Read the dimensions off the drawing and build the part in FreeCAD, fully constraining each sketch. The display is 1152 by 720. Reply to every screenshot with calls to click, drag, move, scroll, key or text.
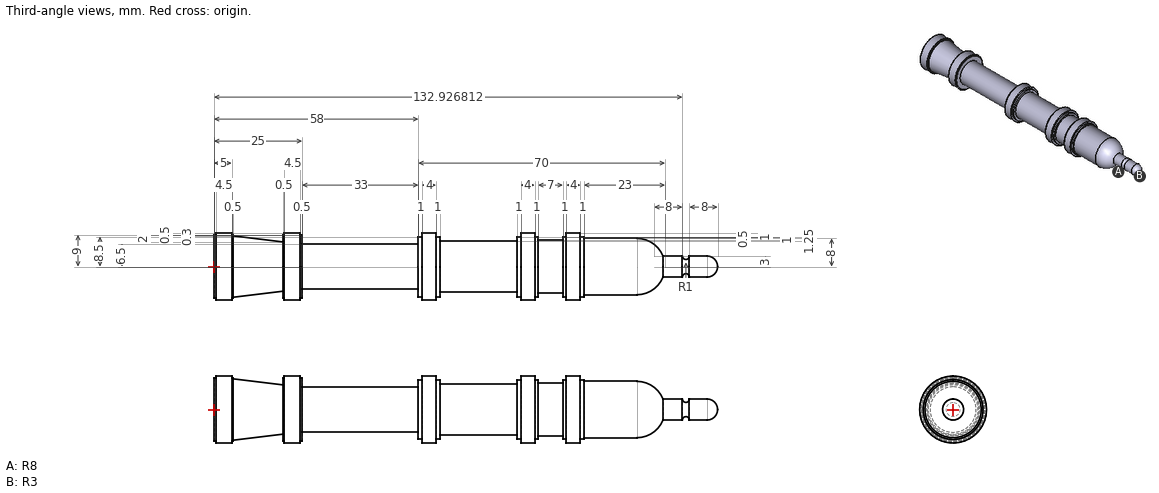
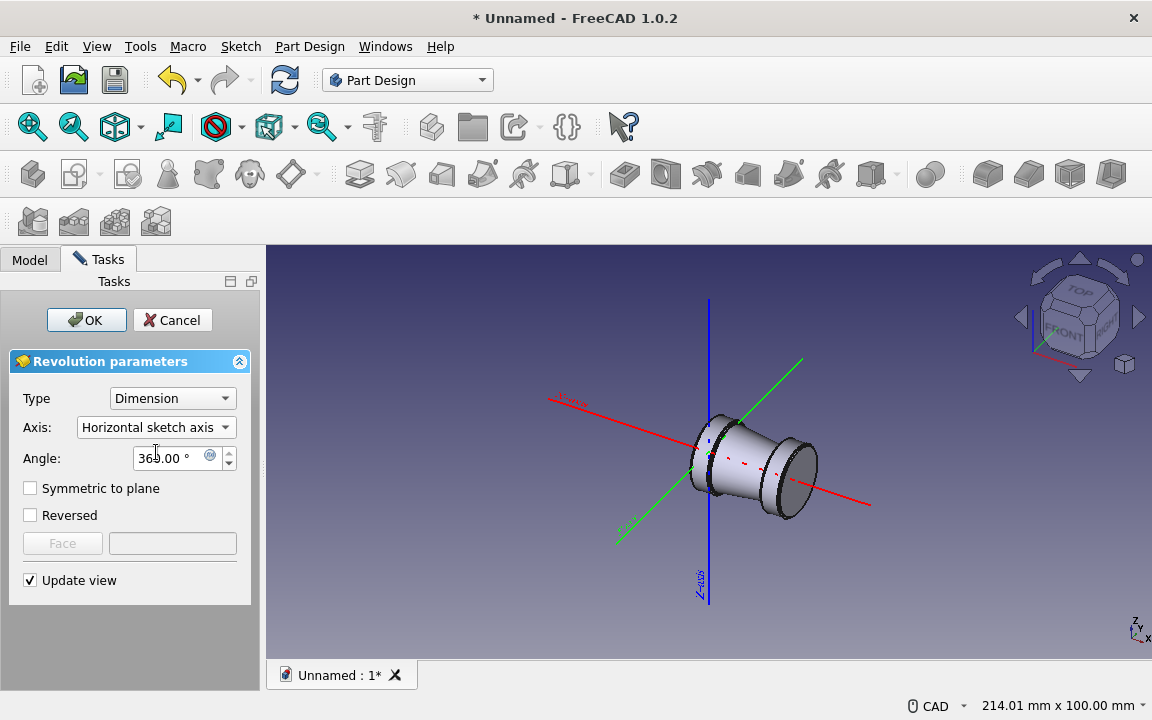
click(87, 320)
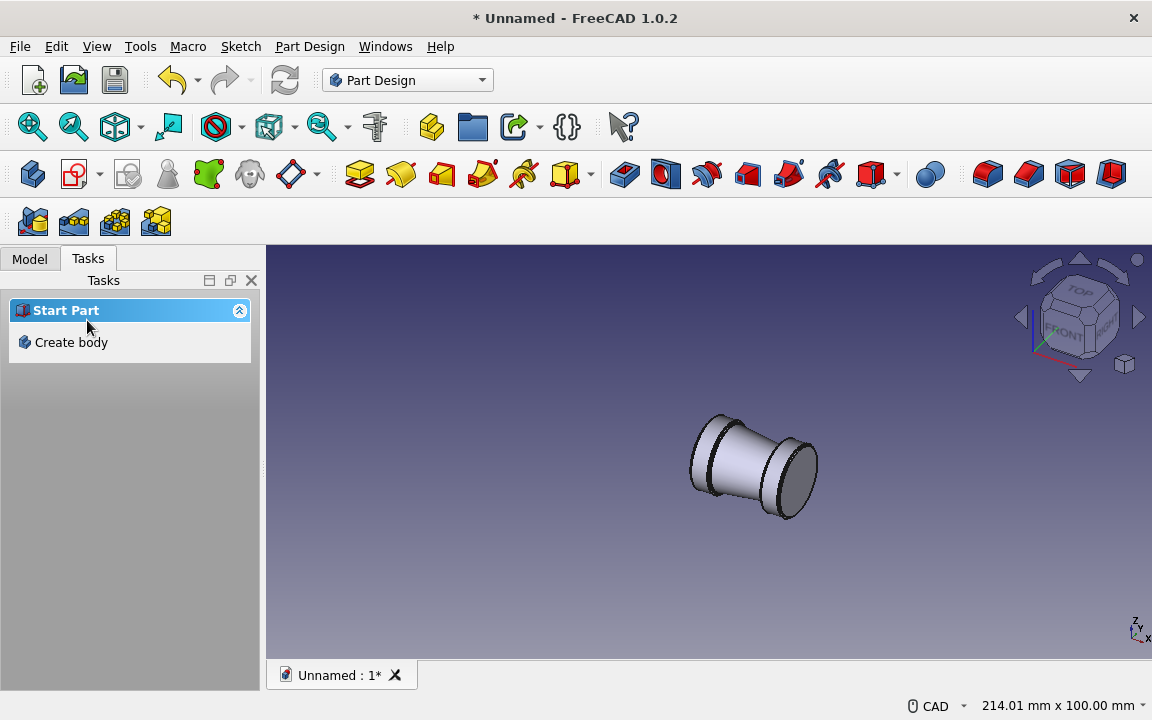
click(33, 128)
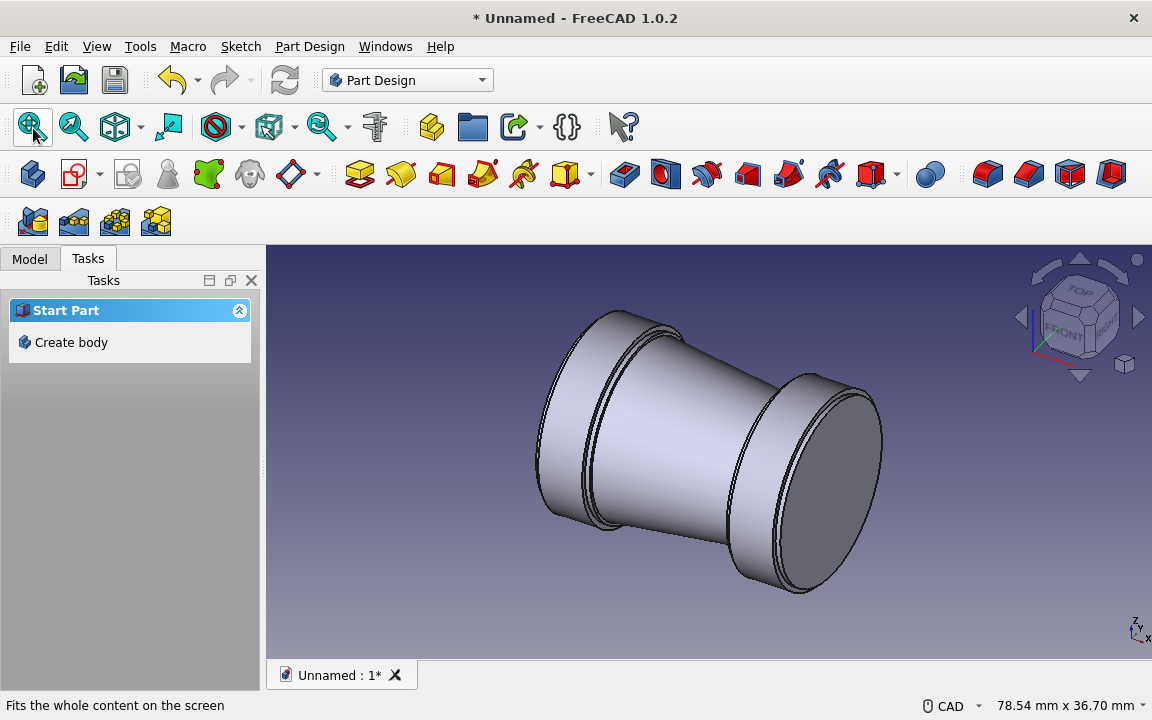
click(74, 174)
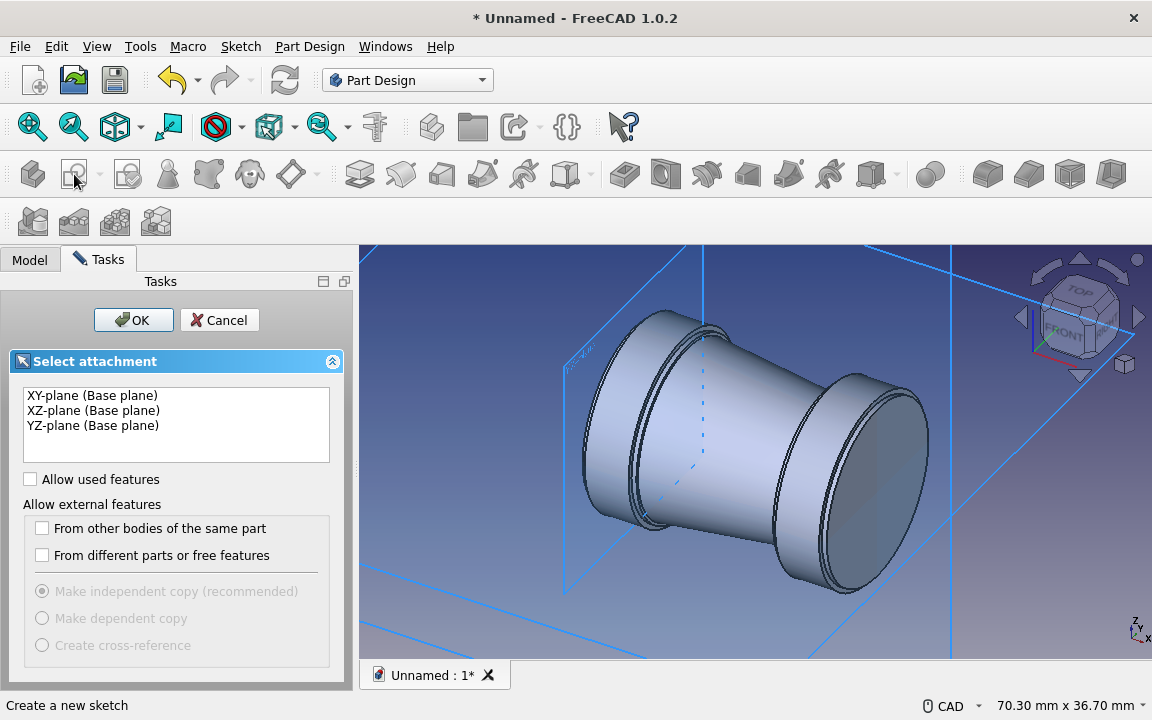
click(84, 396)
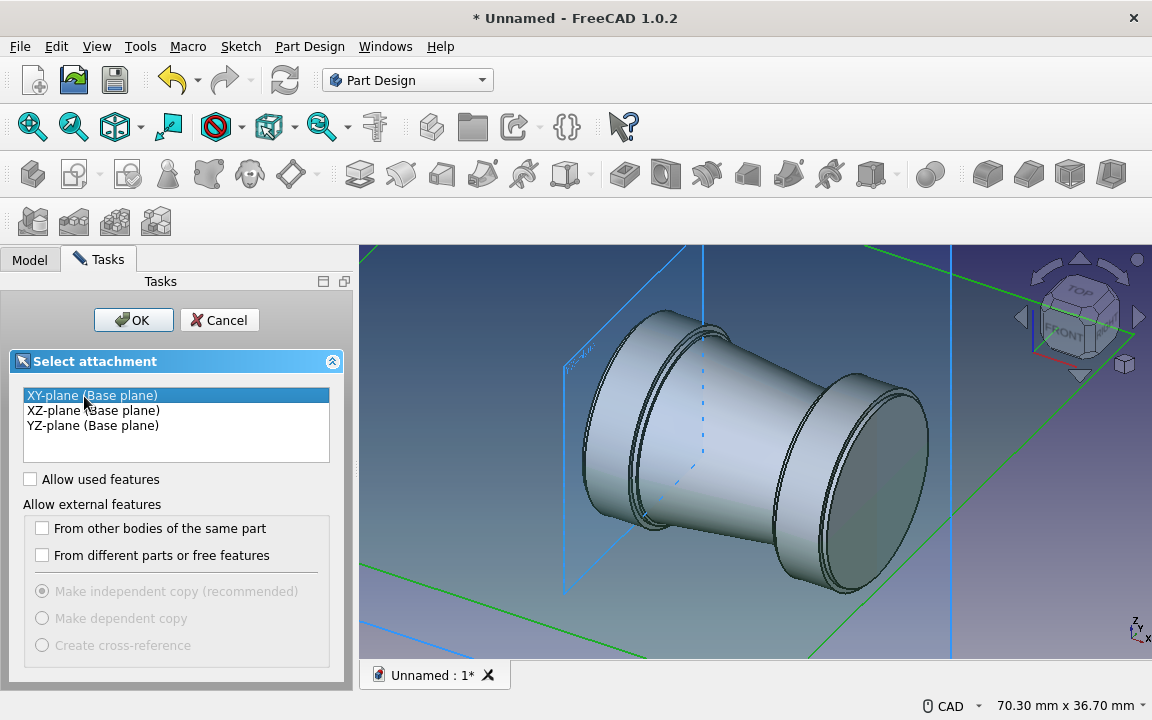
click(134, 320)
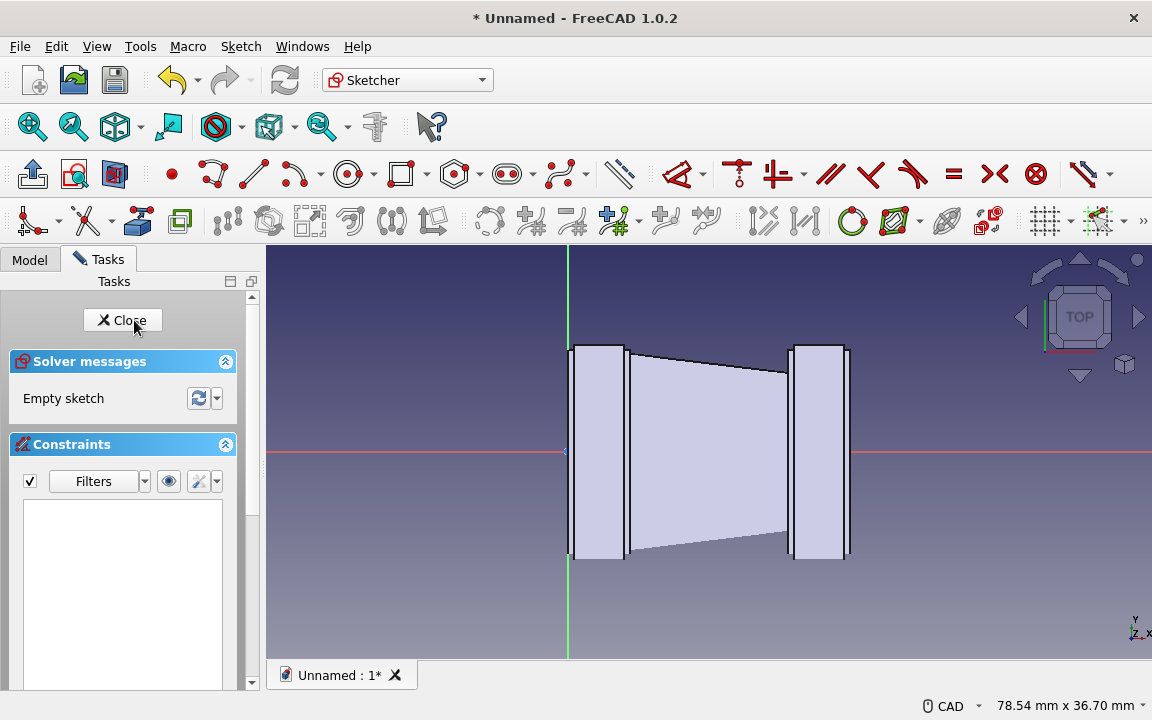
click(115, 174)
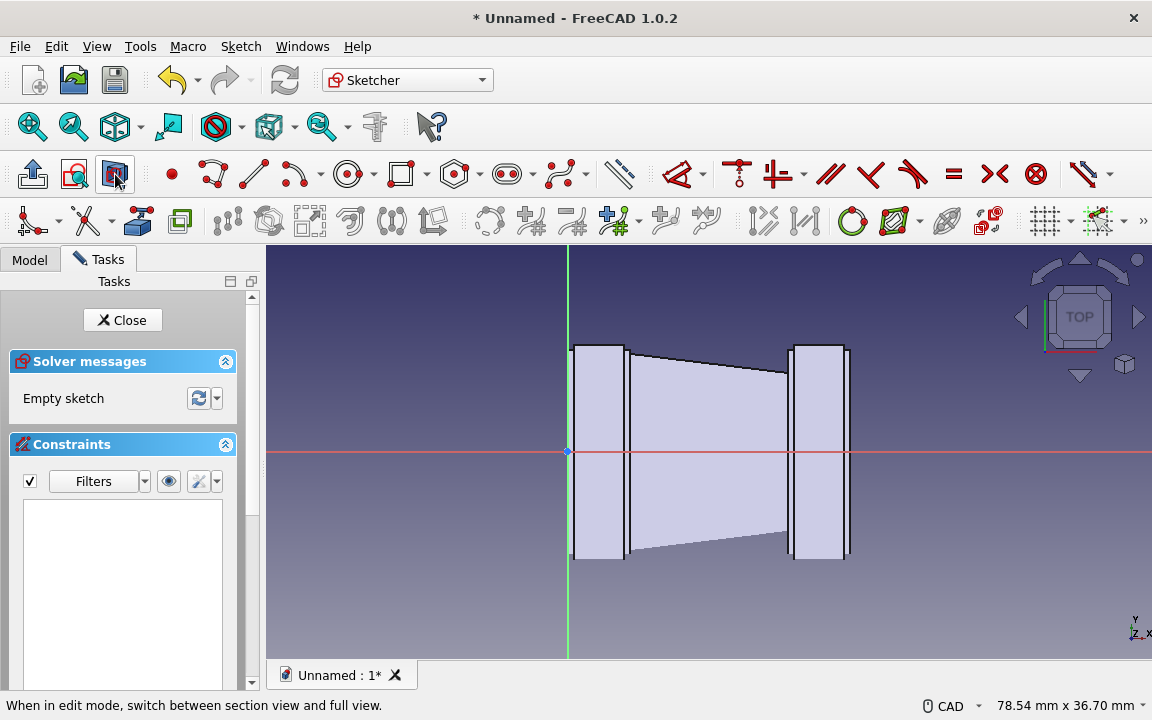
scroll(294, 527, down, 2)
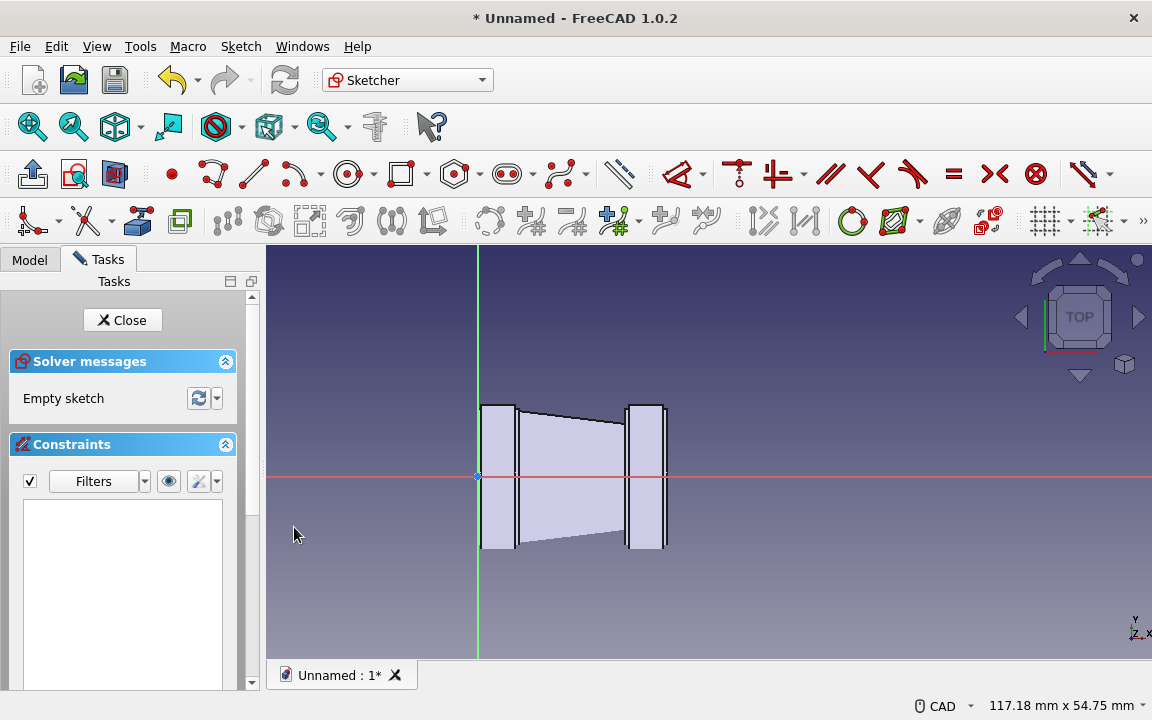
click(400, 174)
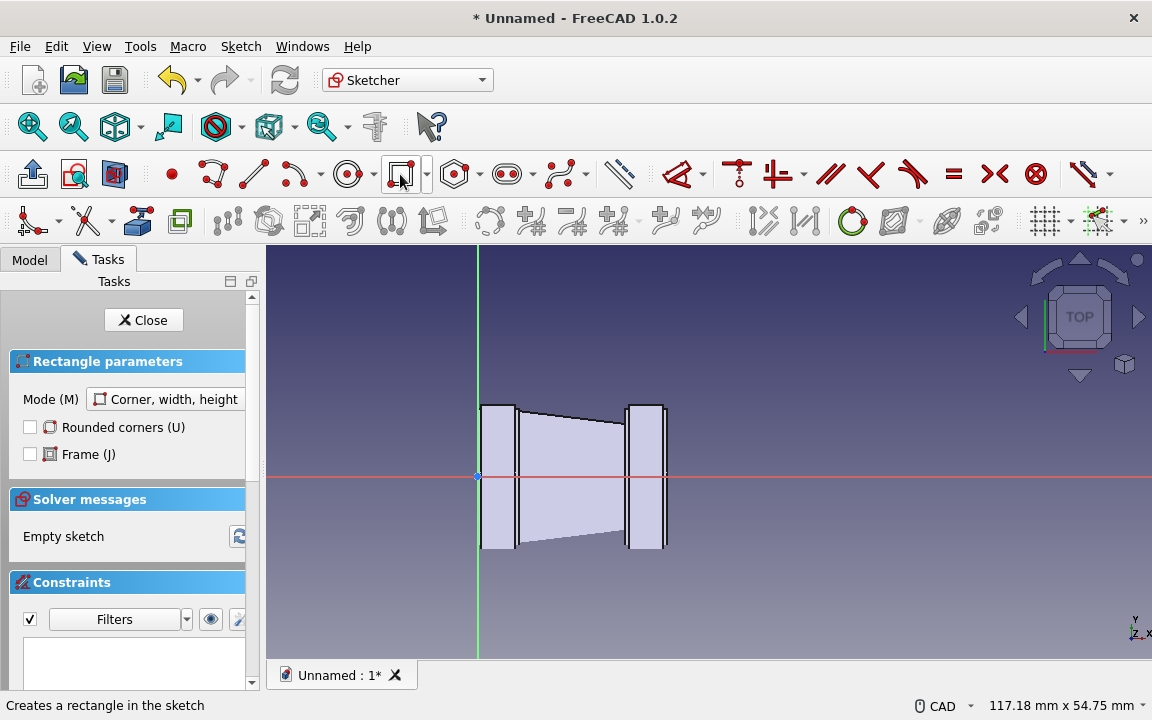
click(667, 428)
click(916, 477)
key(Escape)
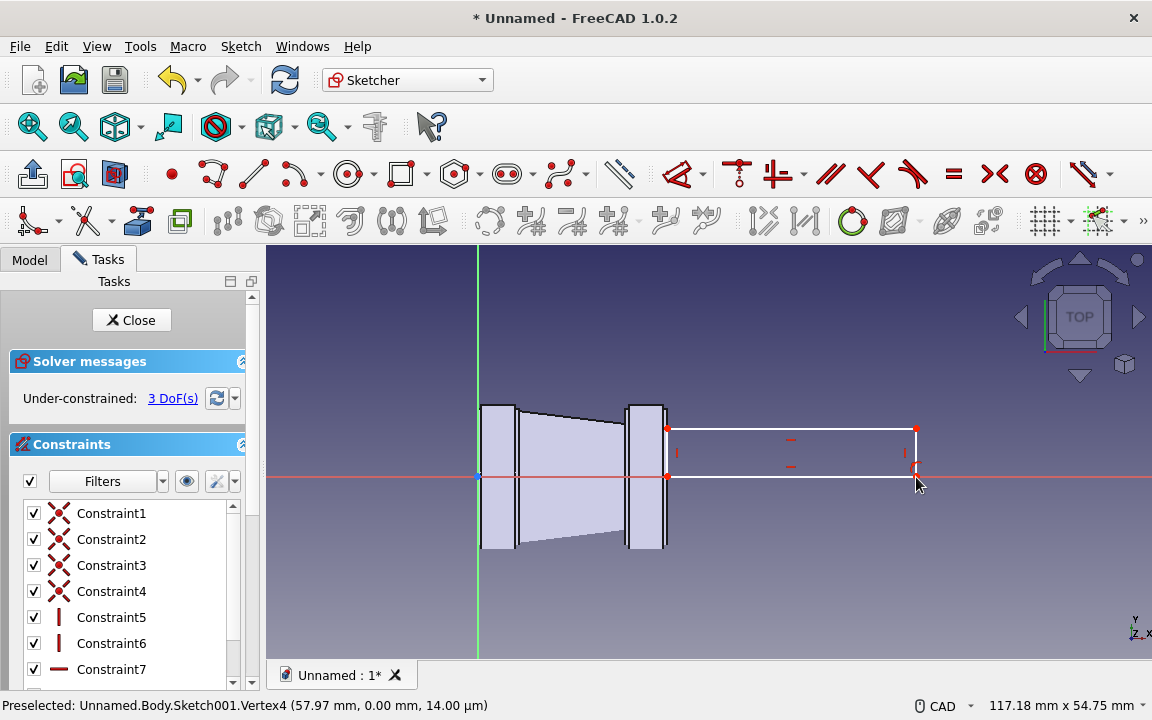
click(676, 174)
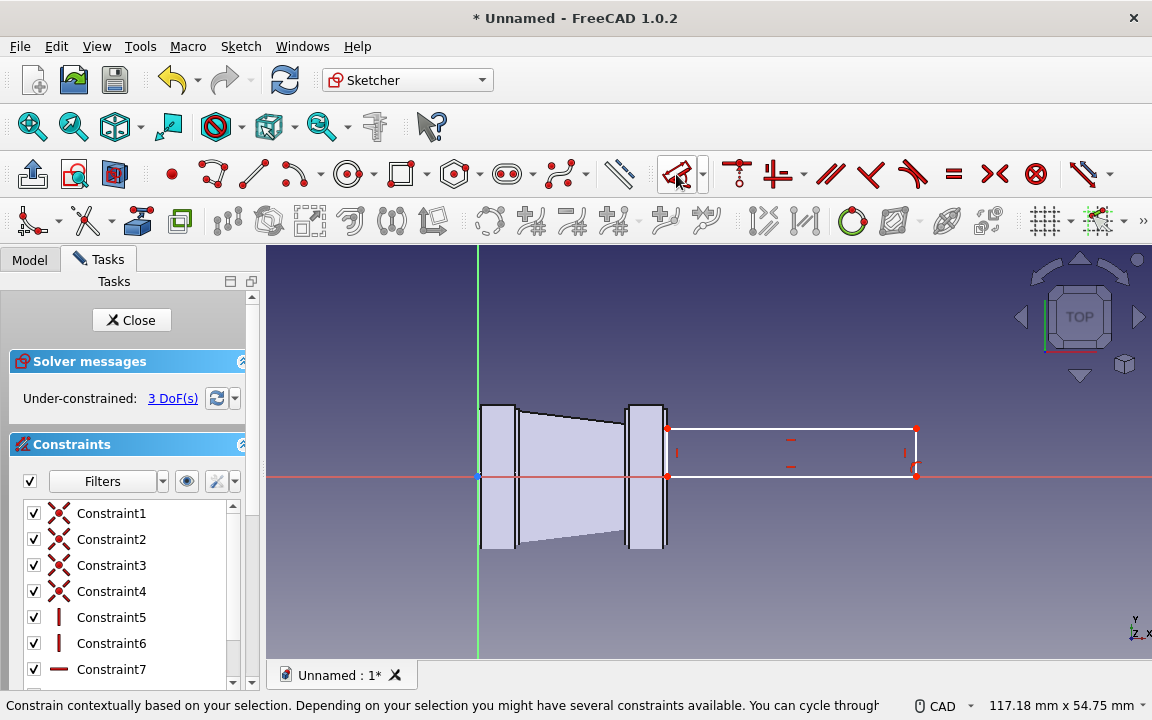
click(742, 477)
click(792, 511)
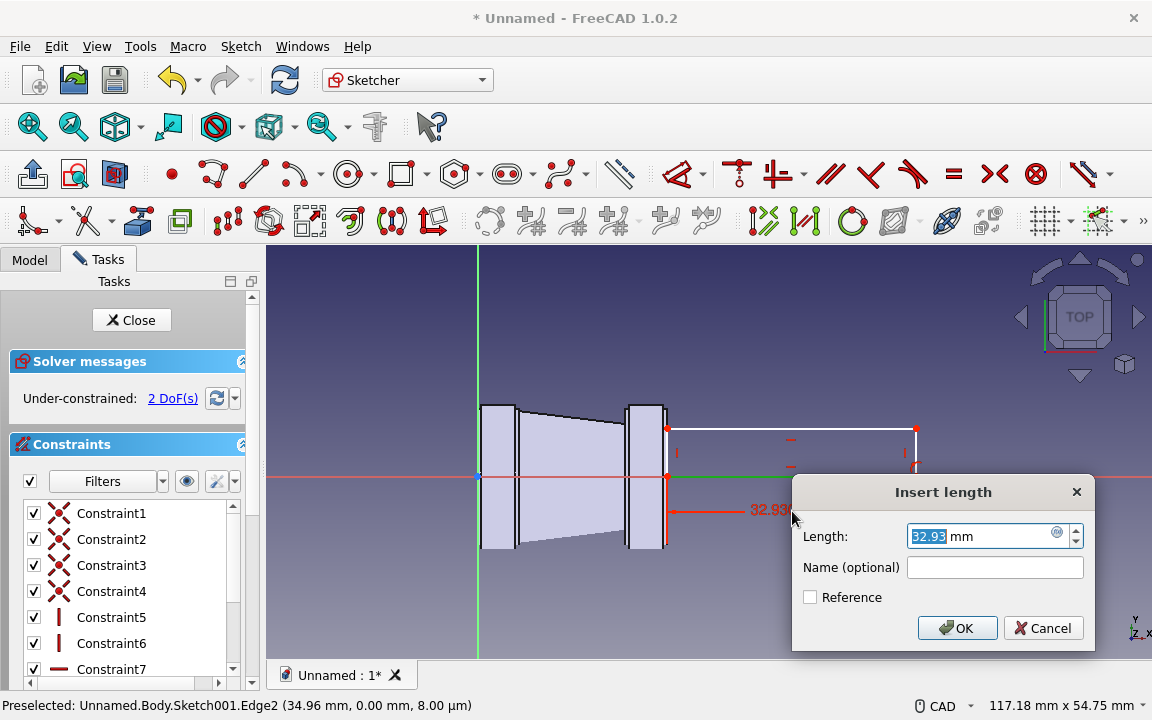
text(33)
key(Return)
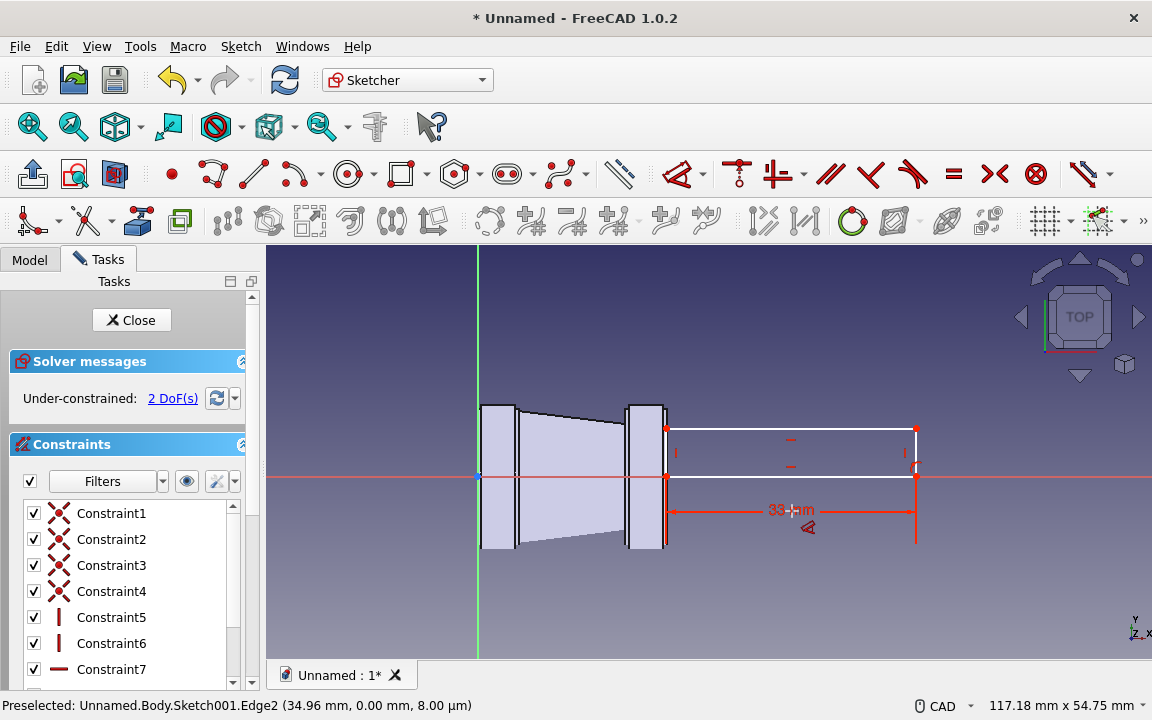
click(666, 443)
click(632, 453)